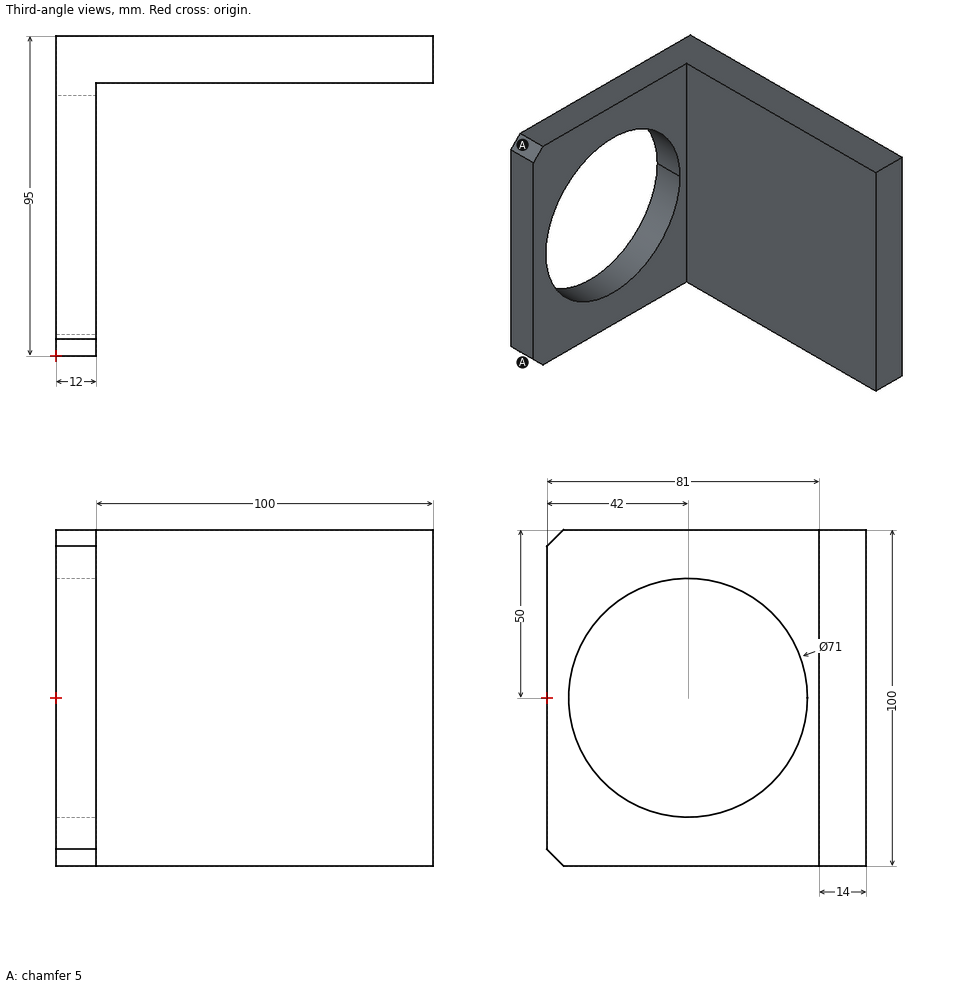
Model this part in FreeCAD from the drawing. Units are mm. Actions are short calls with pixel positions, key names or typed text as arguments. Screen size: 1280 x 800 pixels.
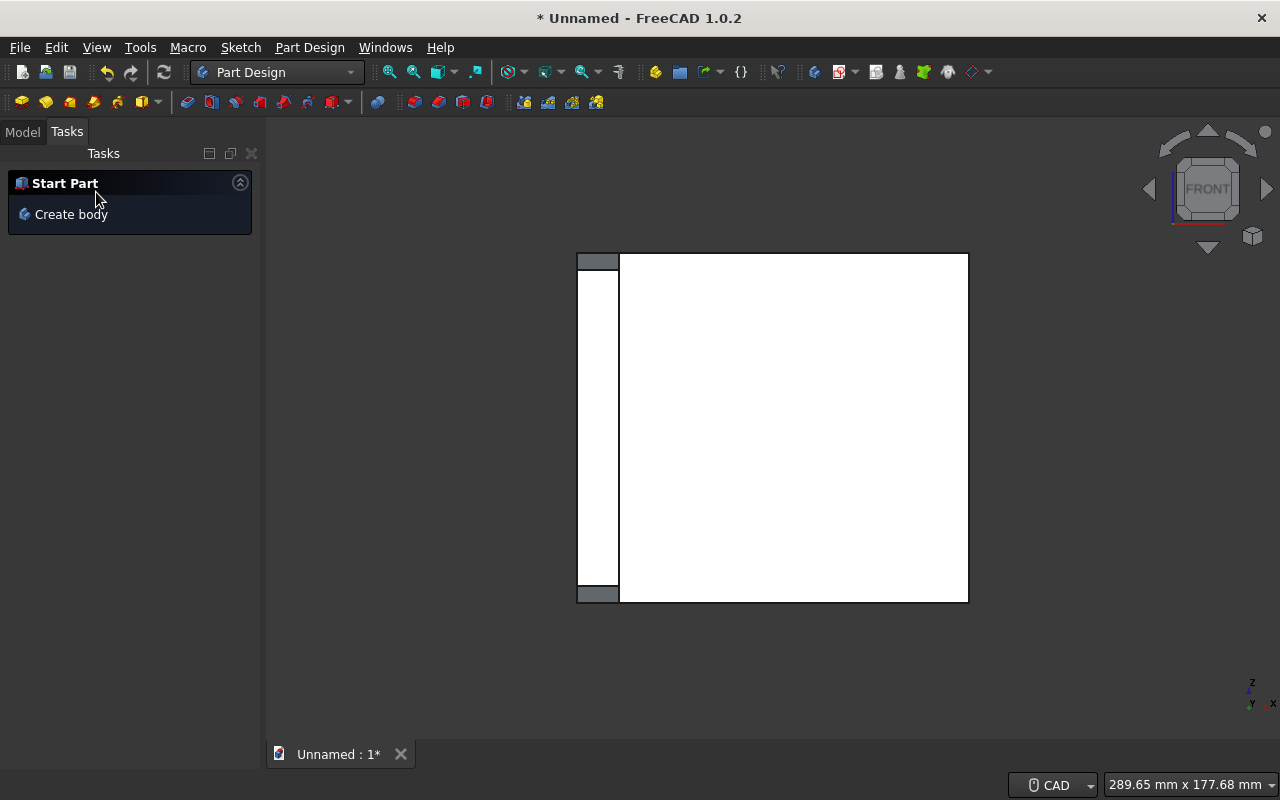
key(0)